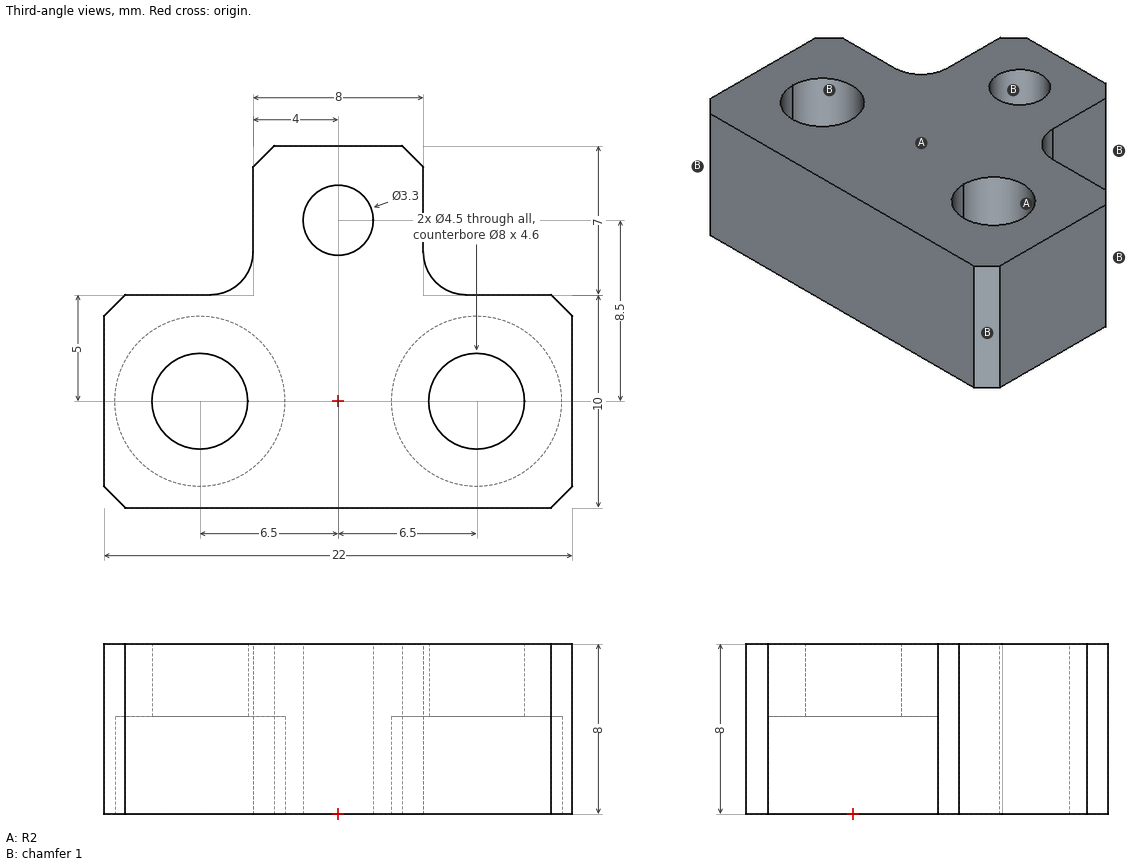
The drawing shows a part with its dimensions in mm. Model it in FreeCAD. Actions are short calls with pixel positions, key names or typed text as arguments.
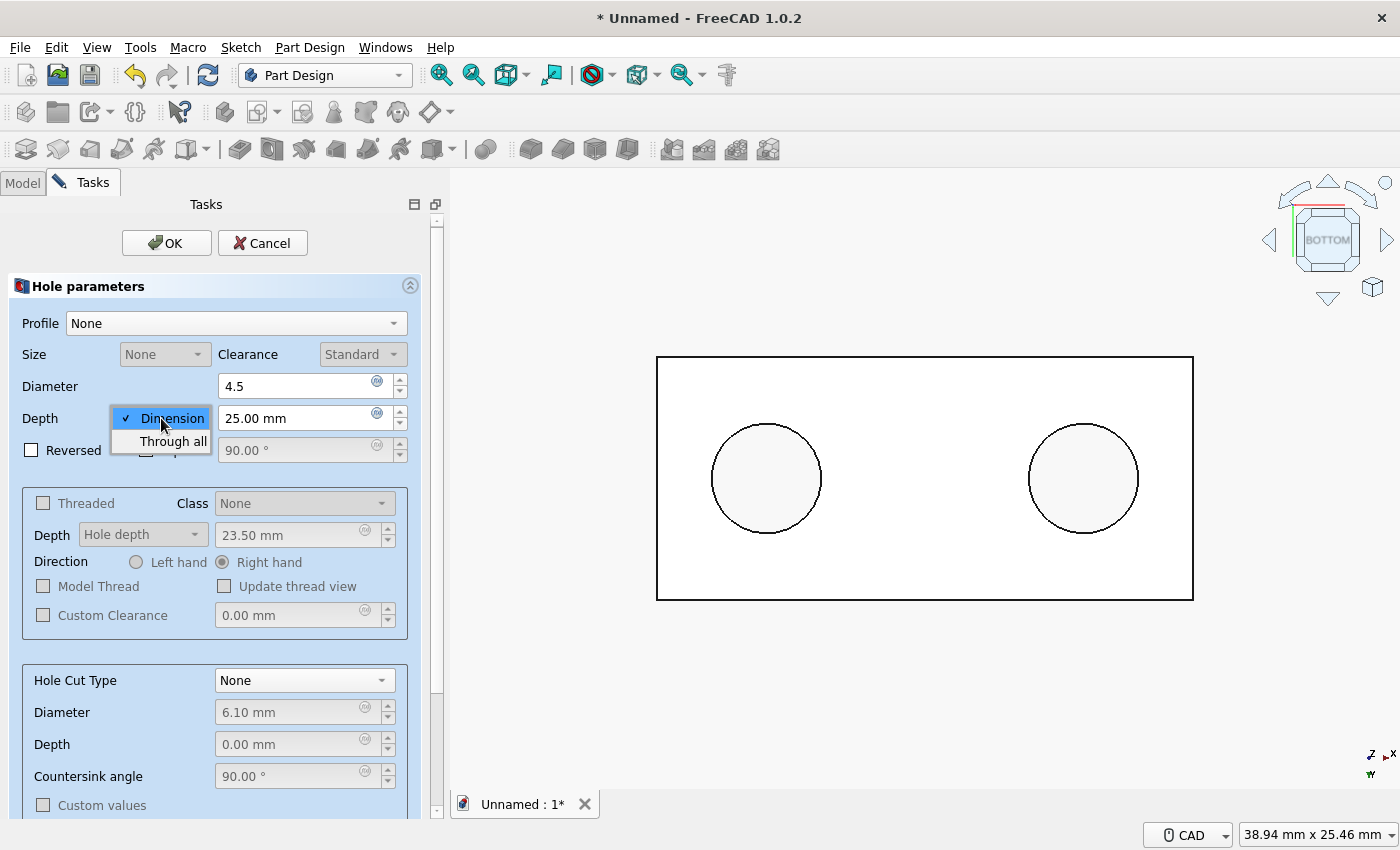
click(160, 442)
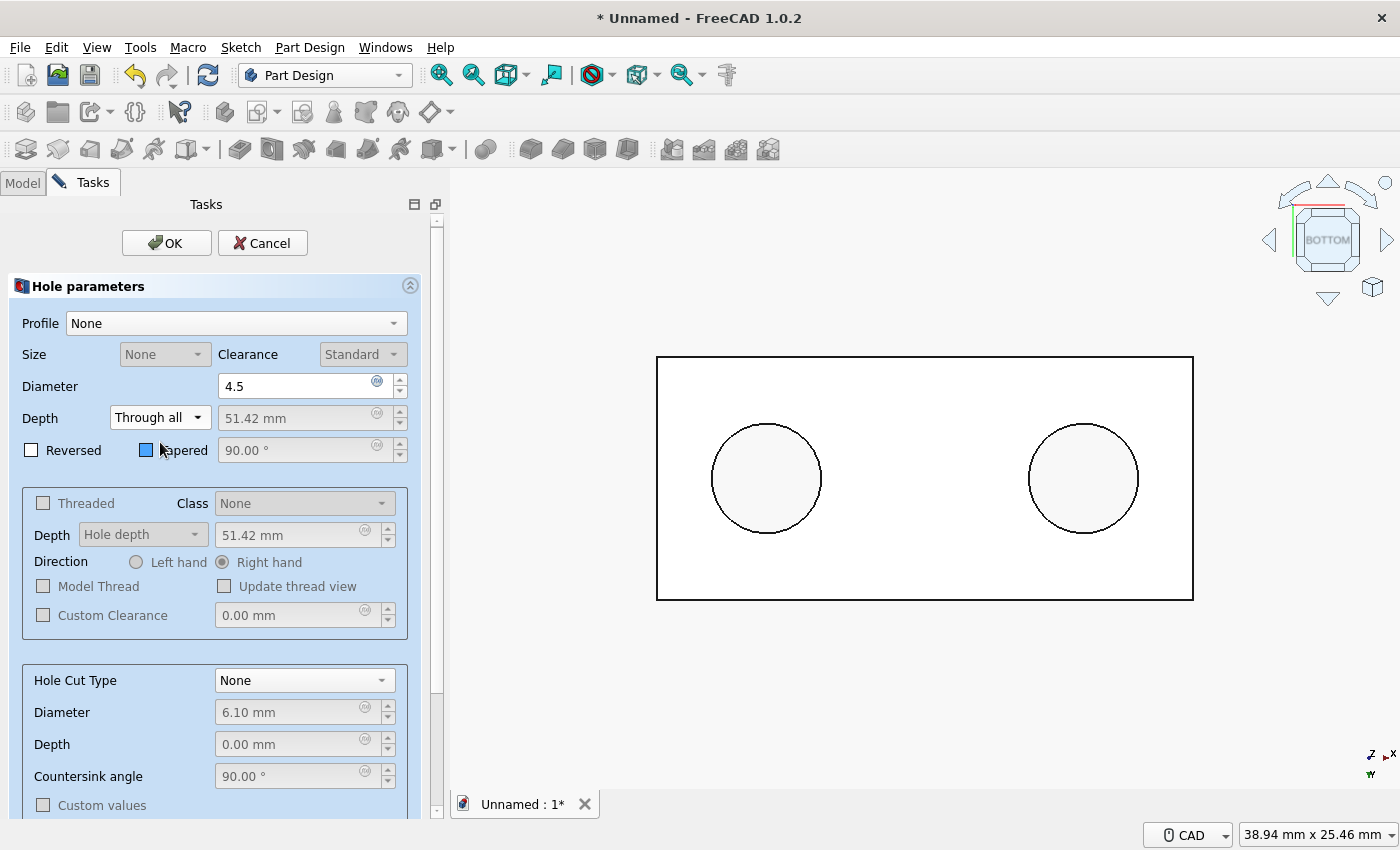
click(306, 680)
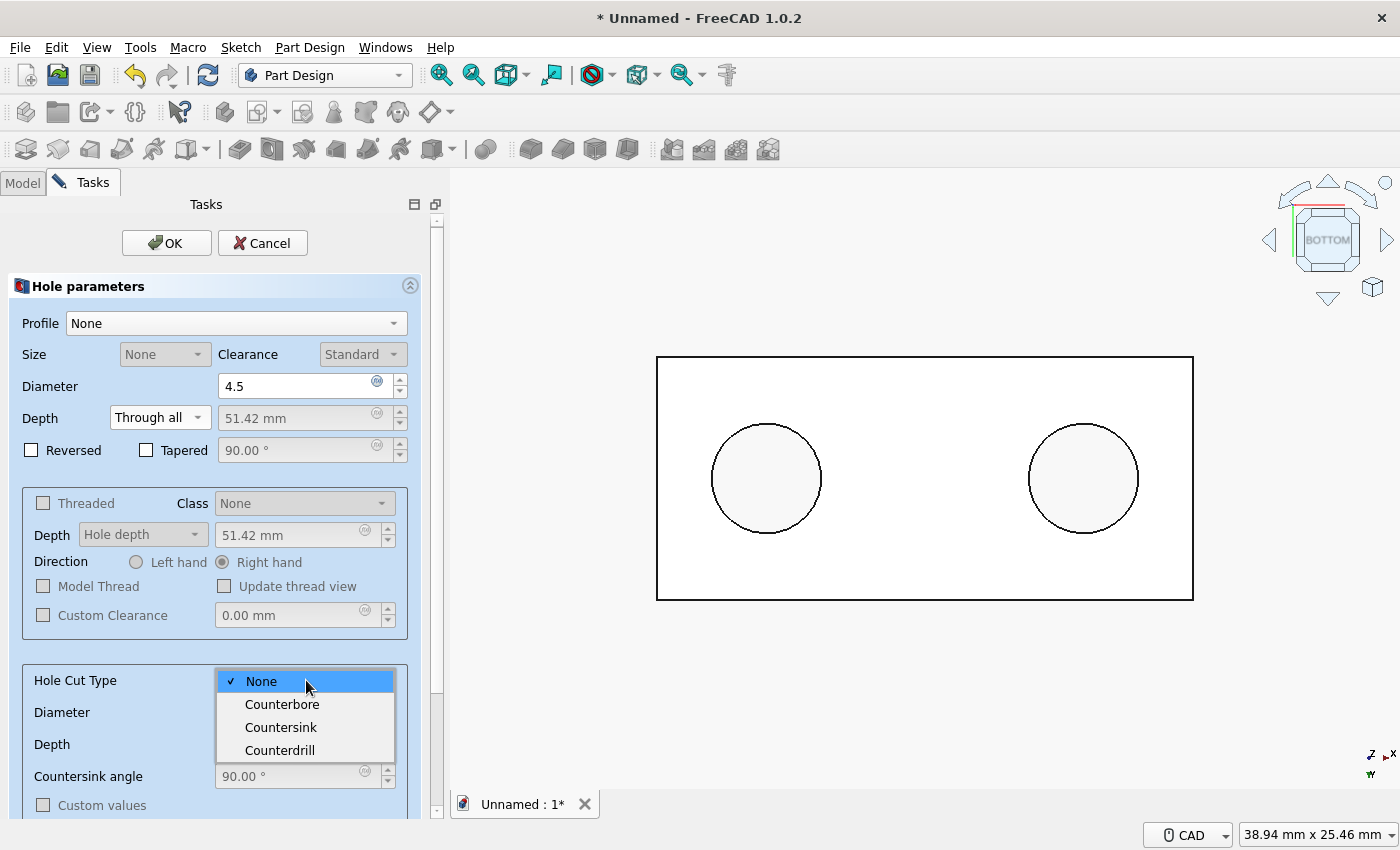
click(304, 704)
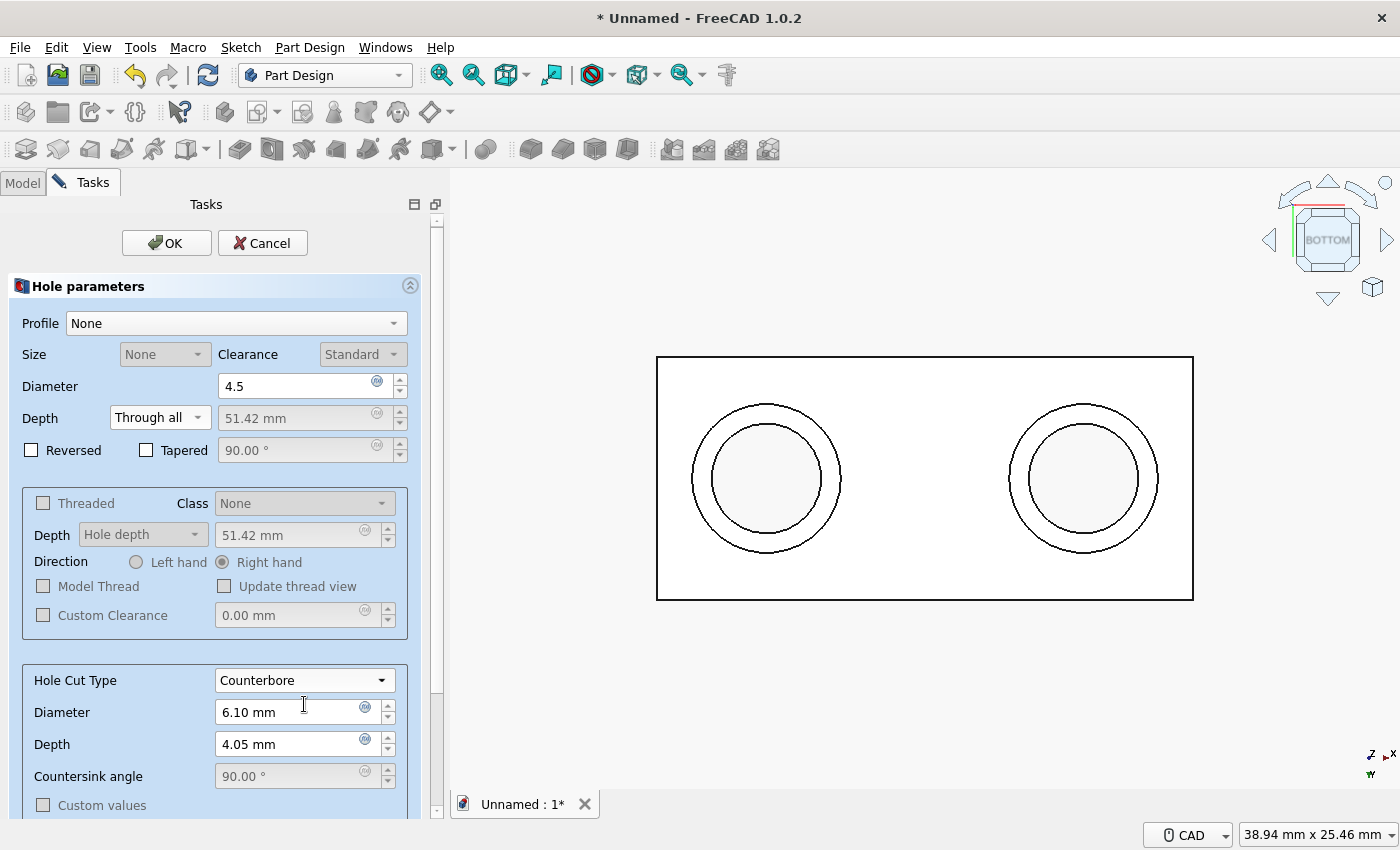
triple_click(298, 712)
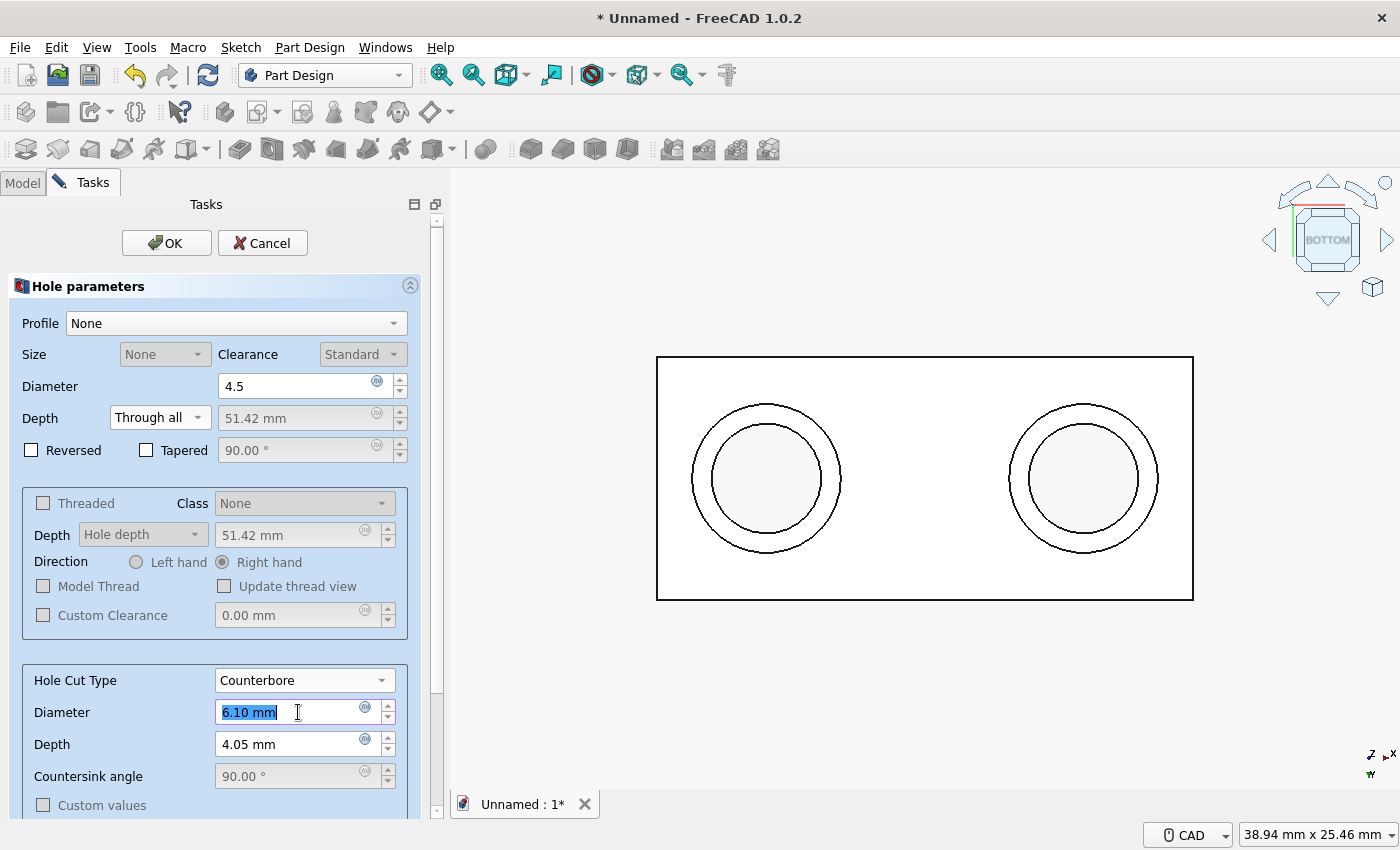
text(8)
key(Tab)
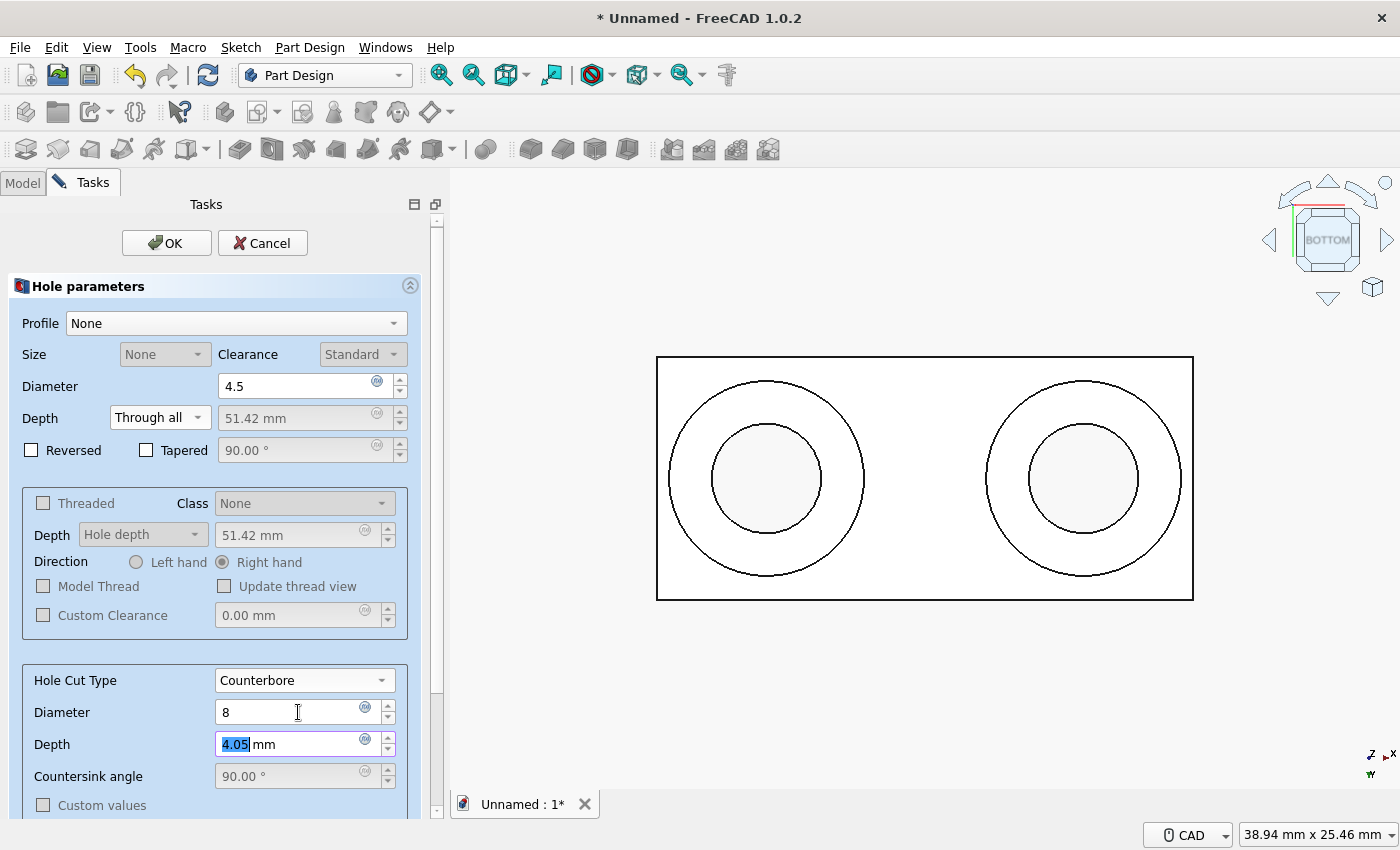
text(4.6)
key(Tab)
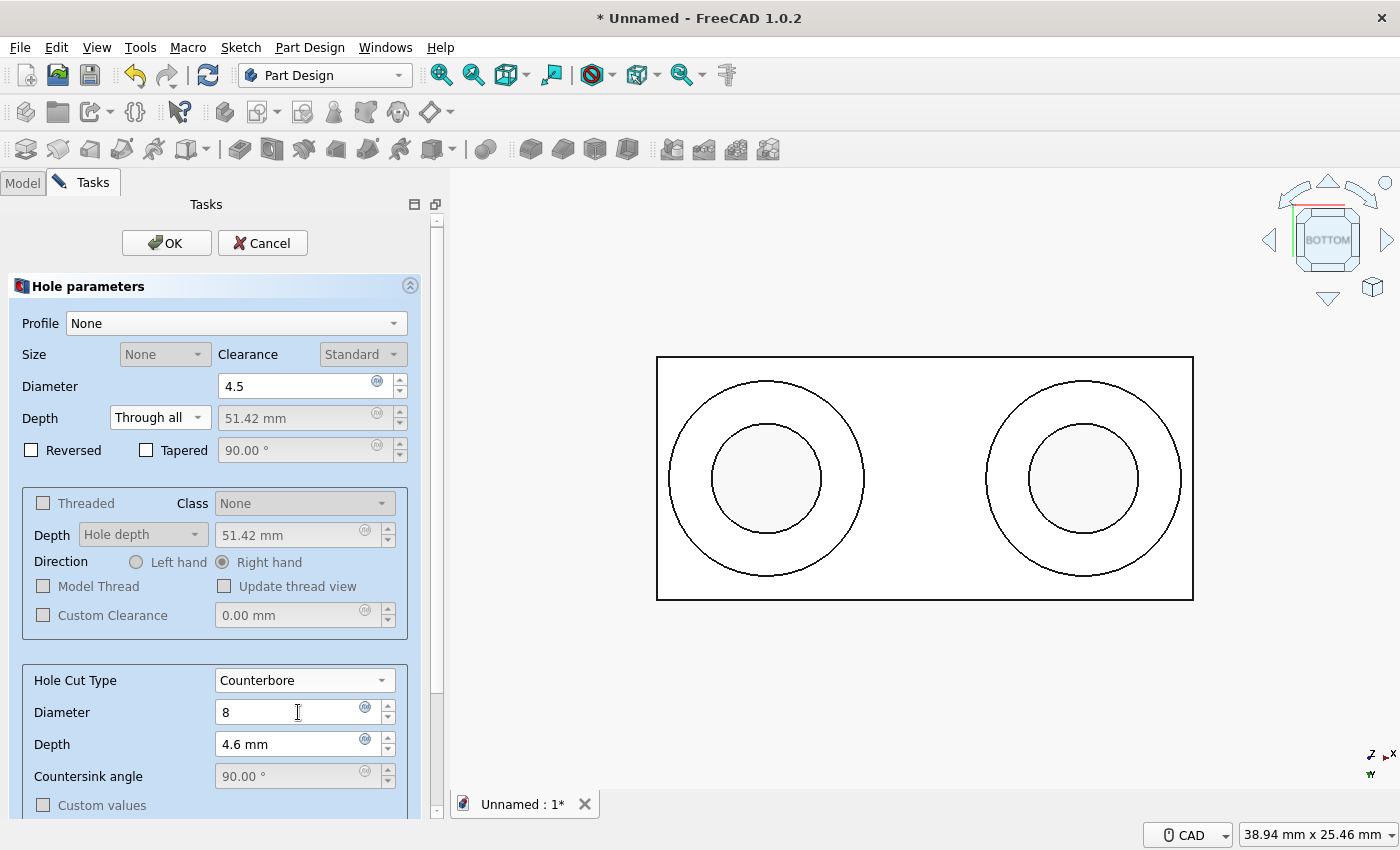
click(167, 243)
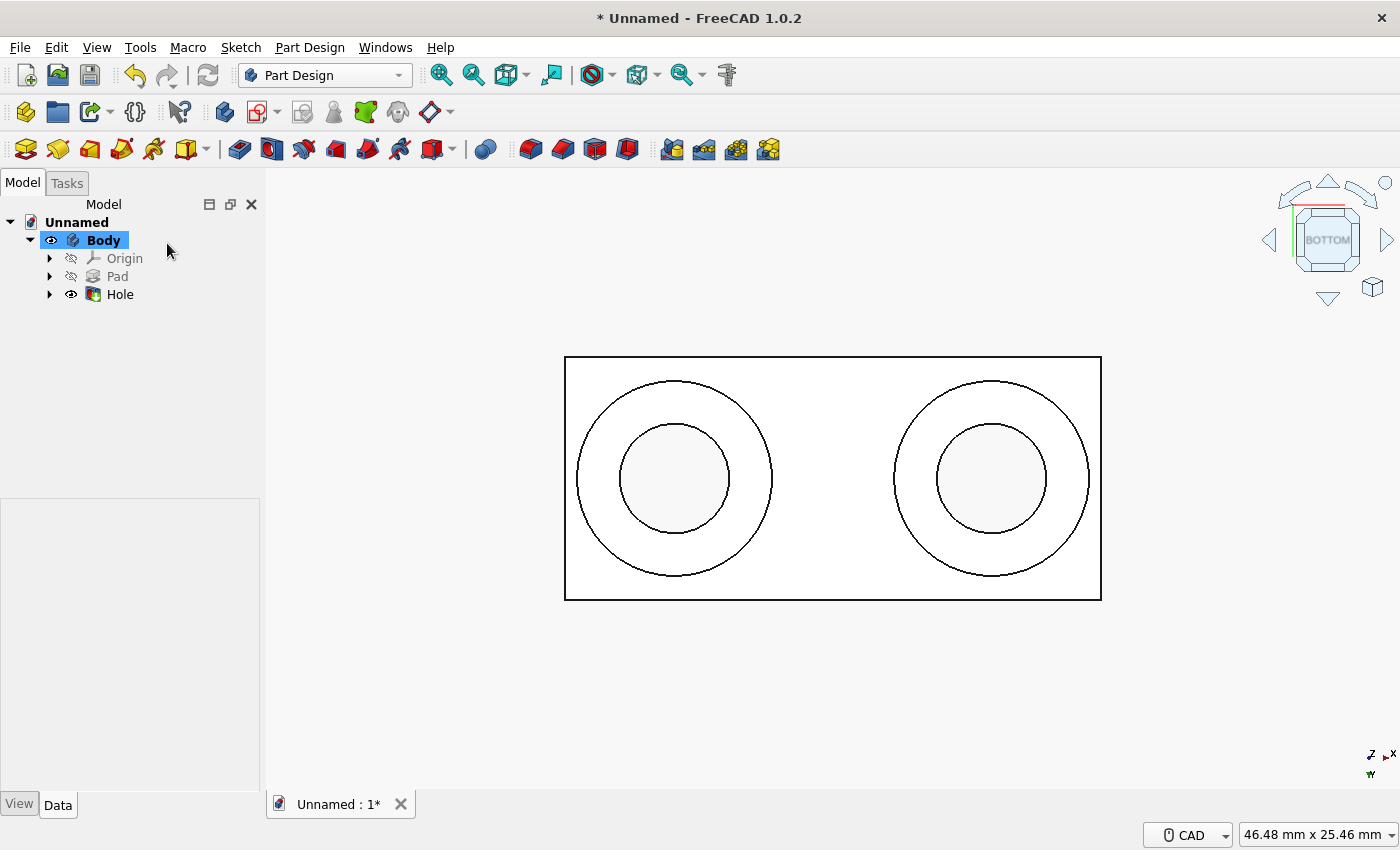
click(258, 112)